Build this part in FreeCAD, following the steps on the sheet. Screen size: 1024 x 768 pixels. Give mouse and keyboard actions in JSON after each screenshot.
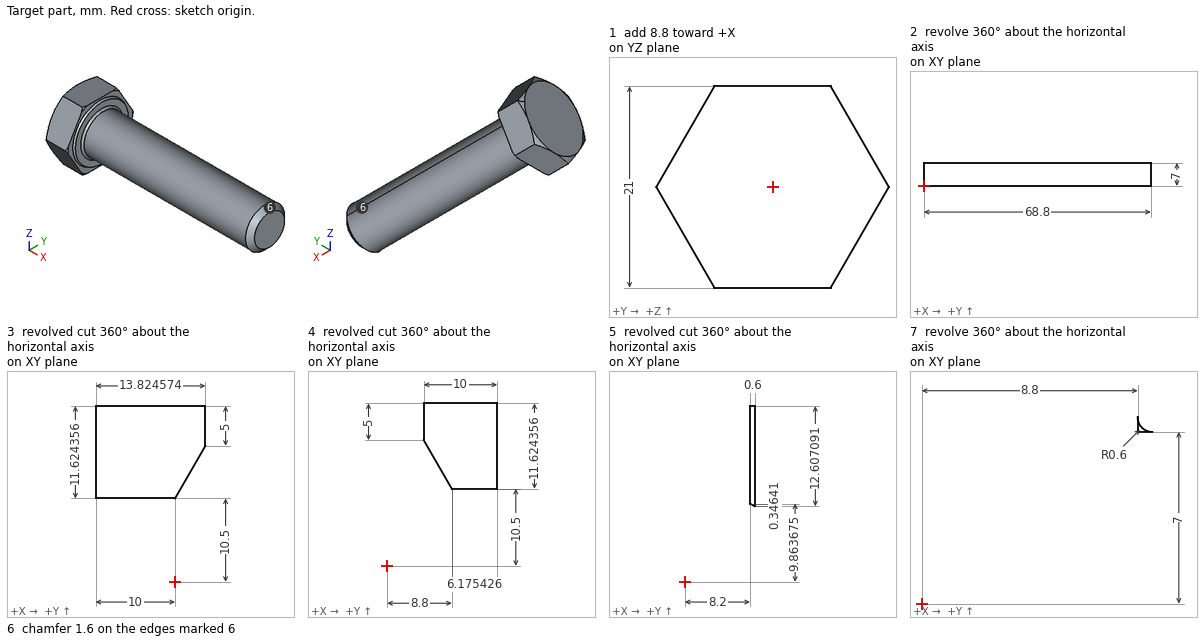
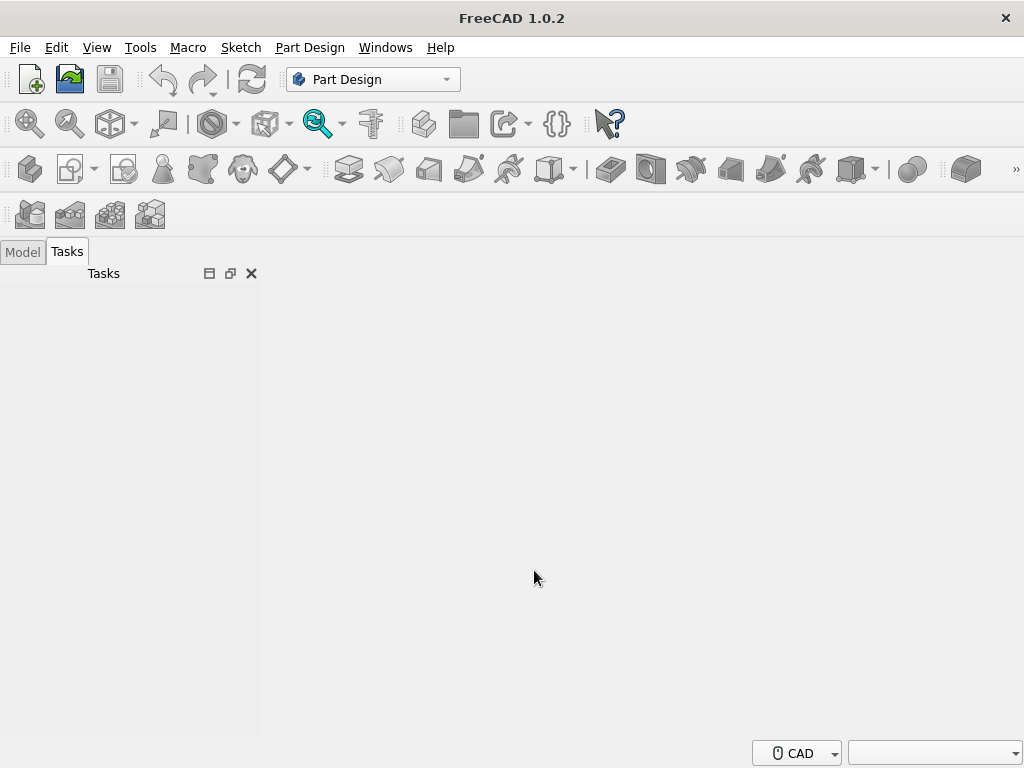
{"action": "left_click", "coordinate": [30, 80]}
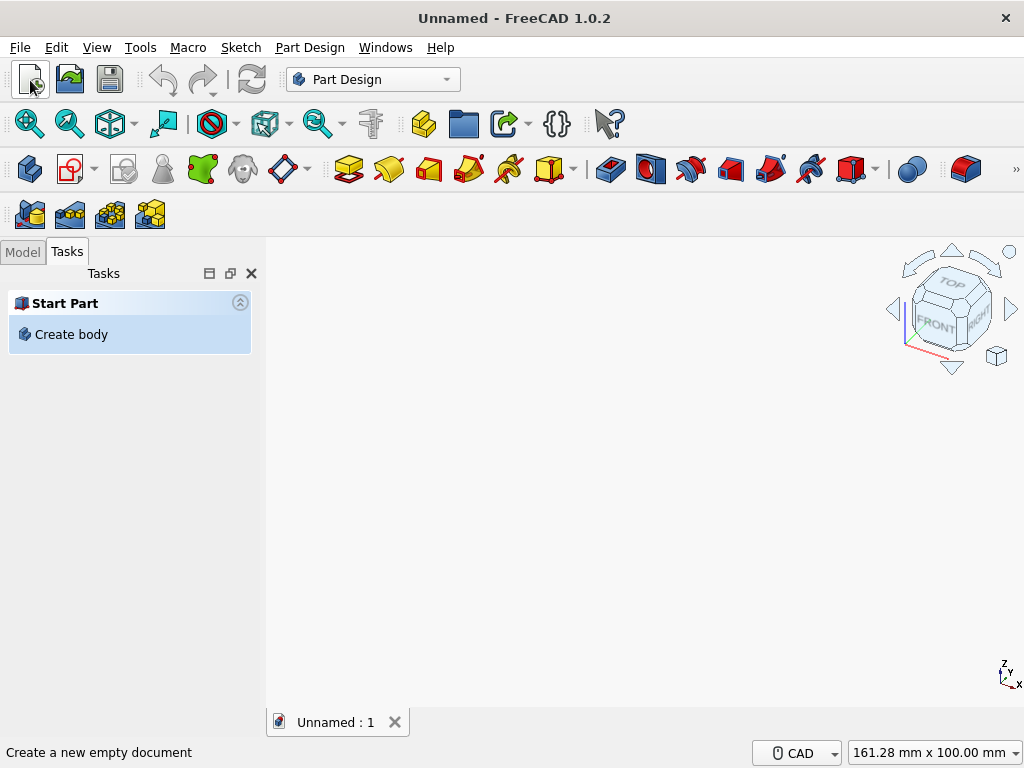
{"action": "left_click", "coordinate": [70, 170]}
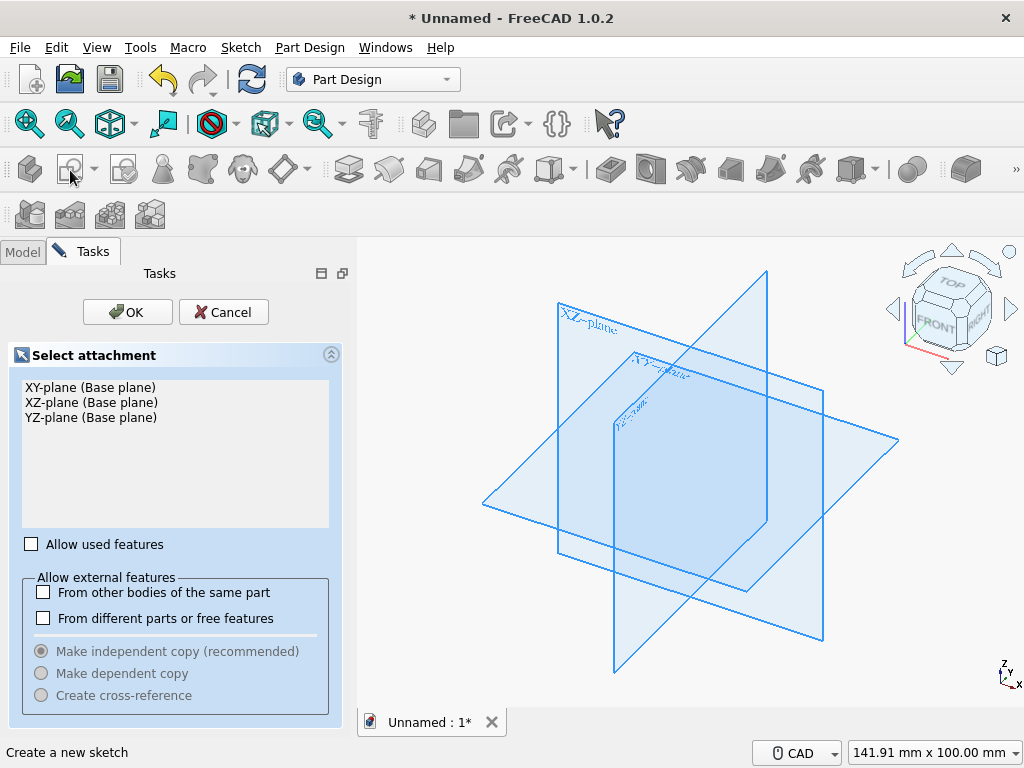
{"action": "left_click", "coordinate": [82, 418]}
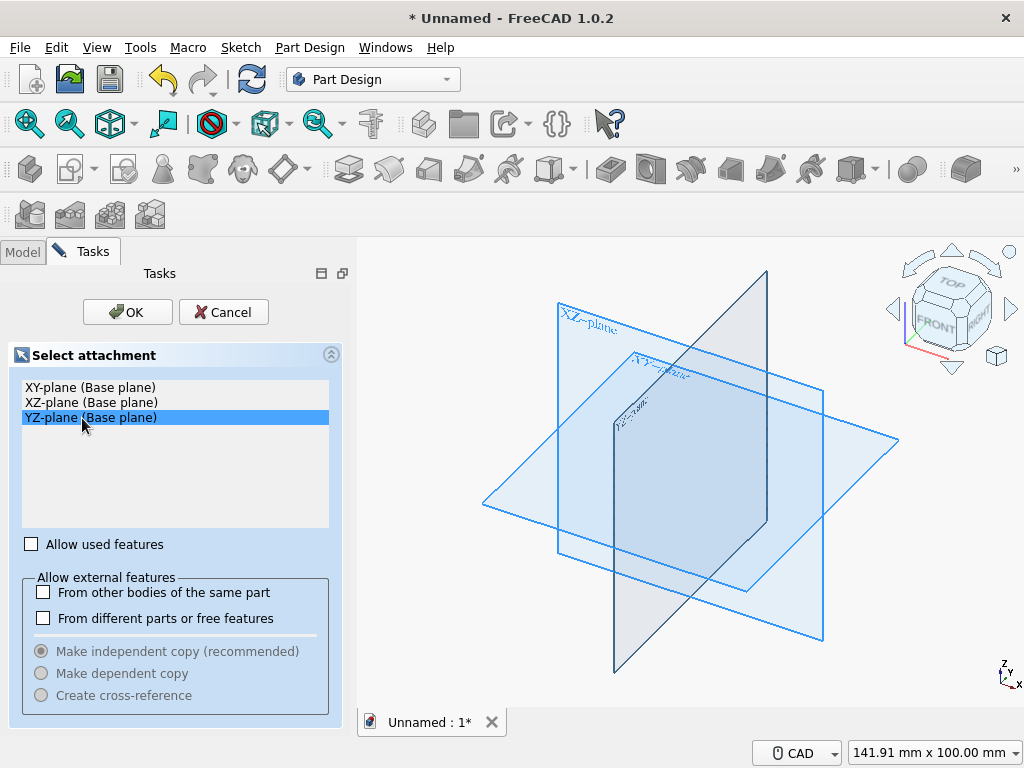
{"action": "left_click", "coordinate": [128, 312]}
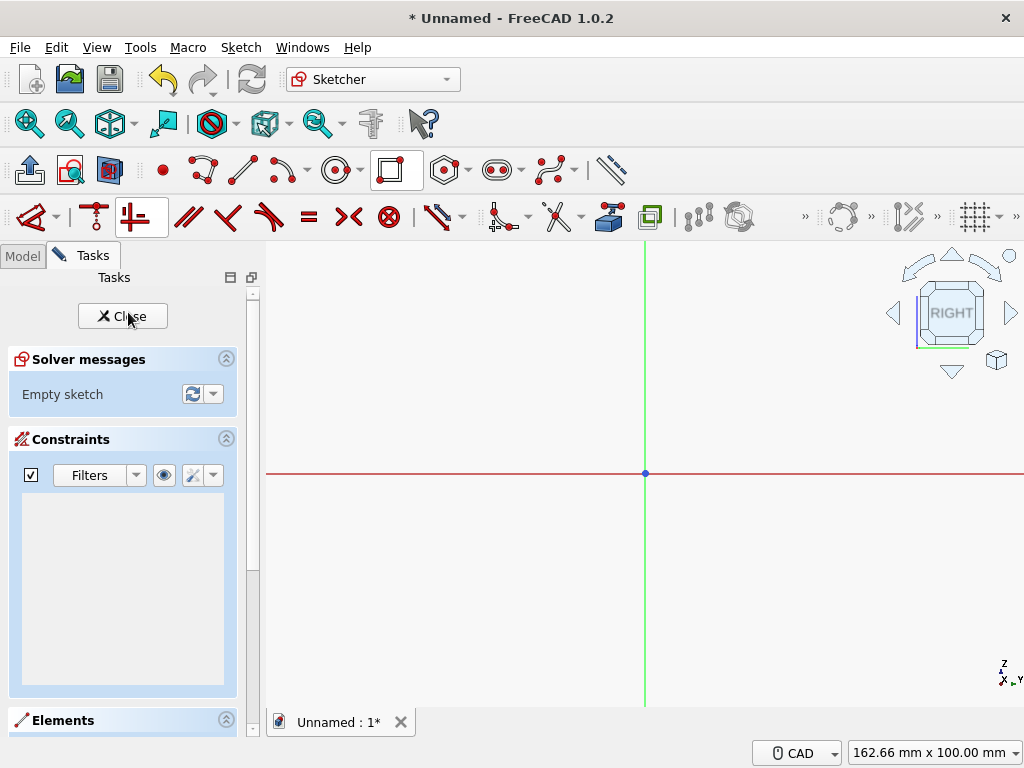
{"action": "scroll", "coordinate": [685, 474], "scroll_direction": "up", "scroll_amount": 5}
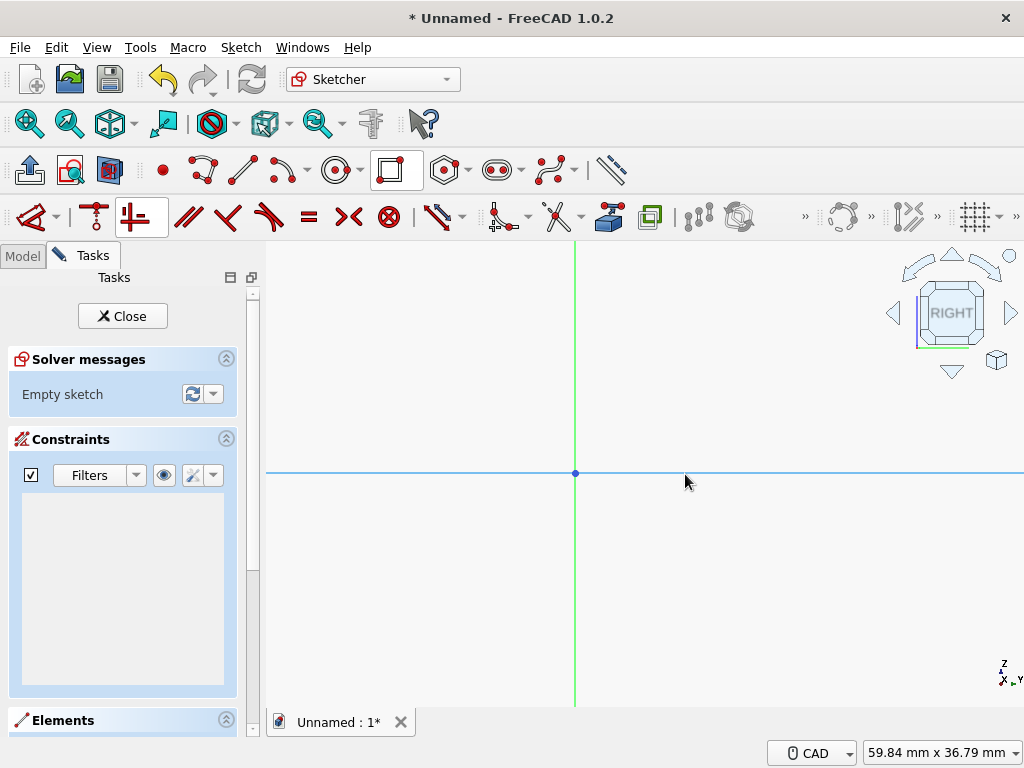
{"action": "left_click", "coordinate": [444, 170]}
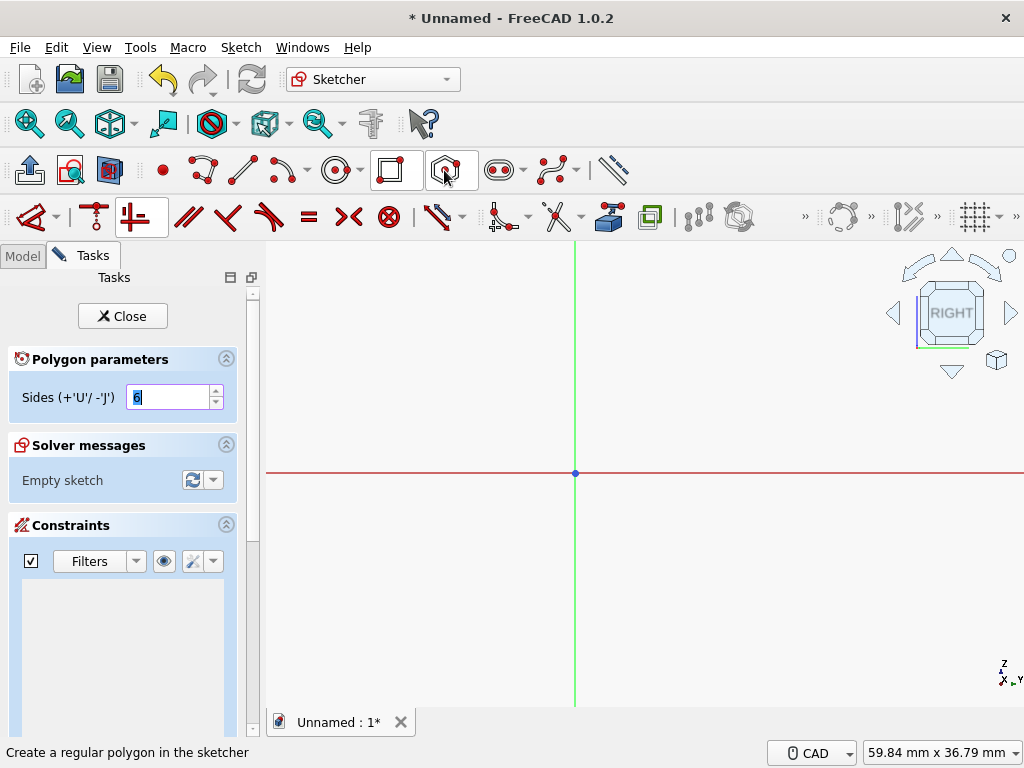
{"action": "left_click", "coordinate": [575, 473]}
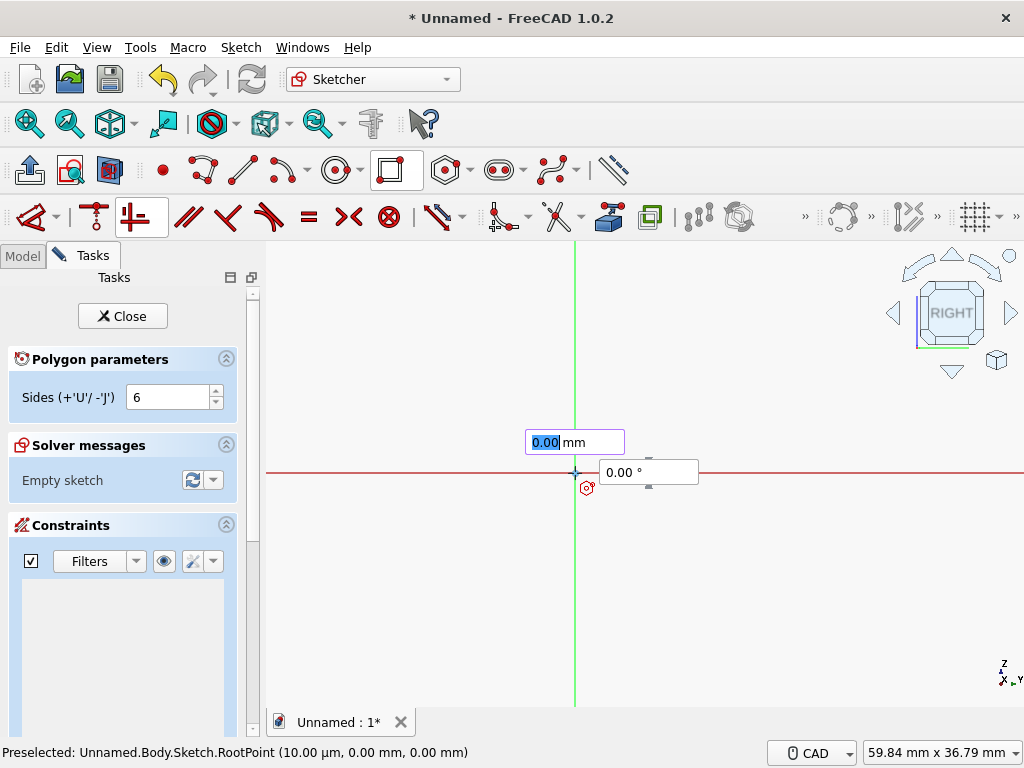
{"action": "left_click", "coordinate": [729, 473]}
{"action": "right_click", "coordinate": [729, 473]}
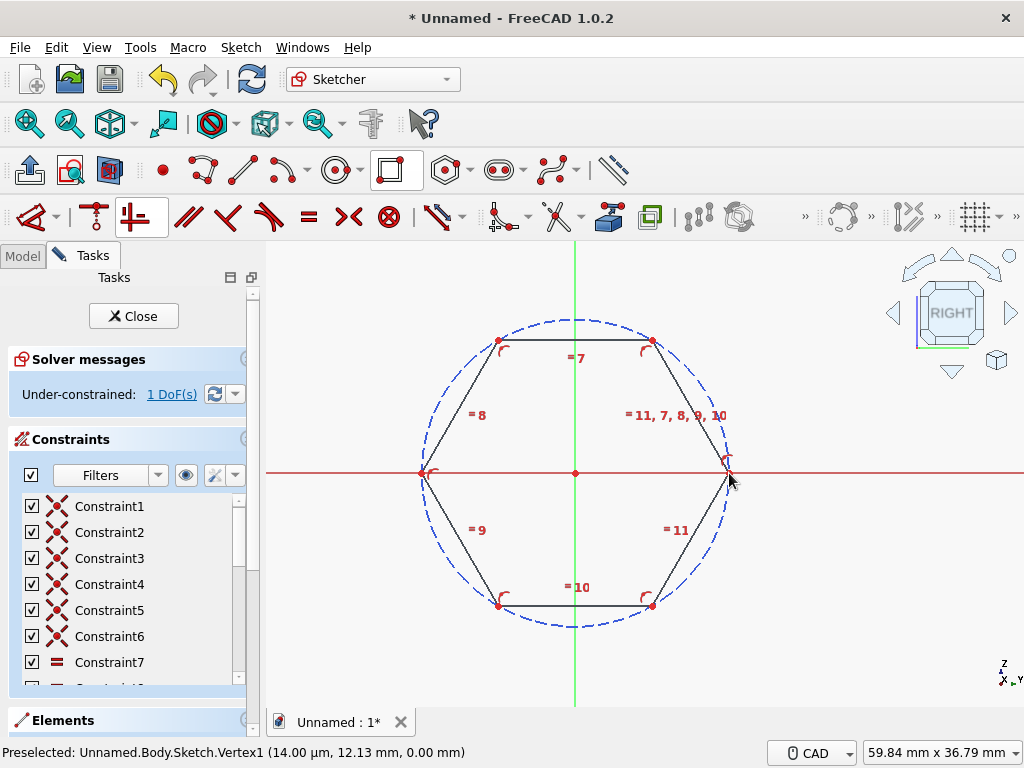
{"action": "left_click", "coordinate": [498, 606]}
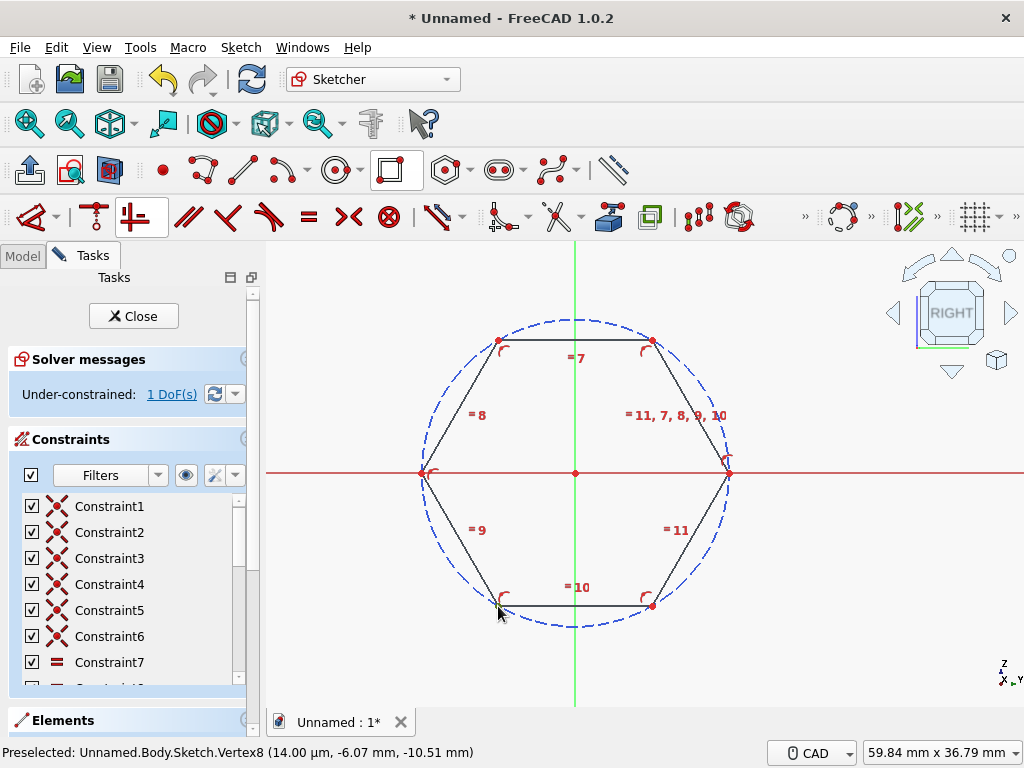
{"action": "left_click", "coordinate": [652, 340]}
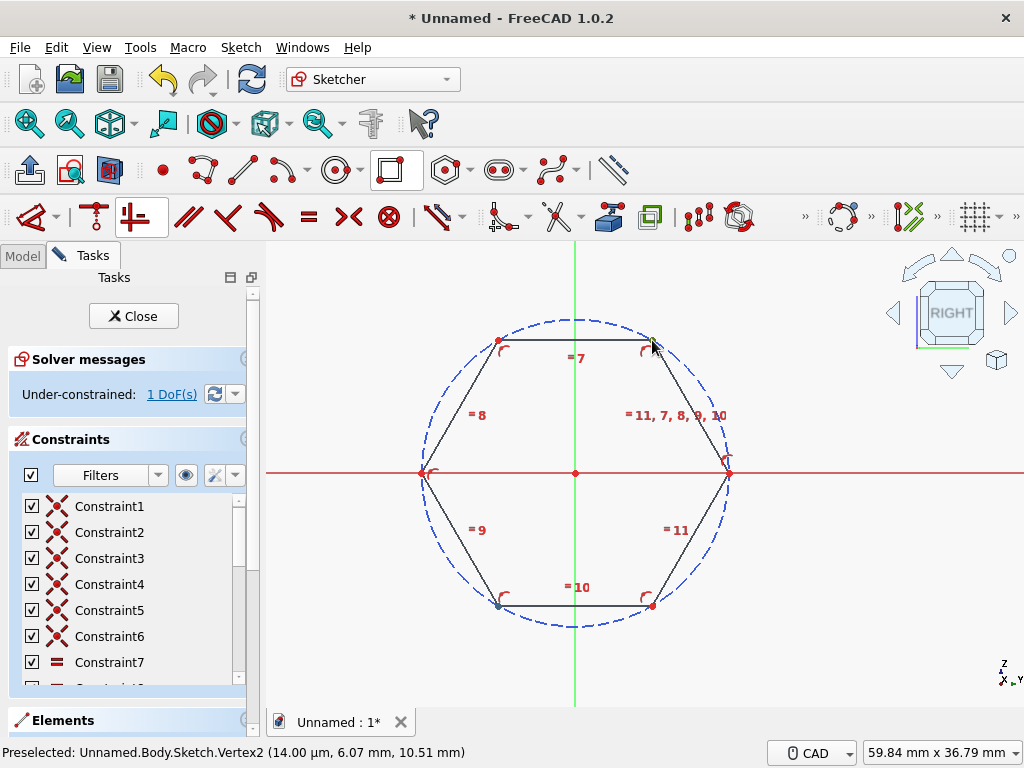
{"action": "key", "text": "i"}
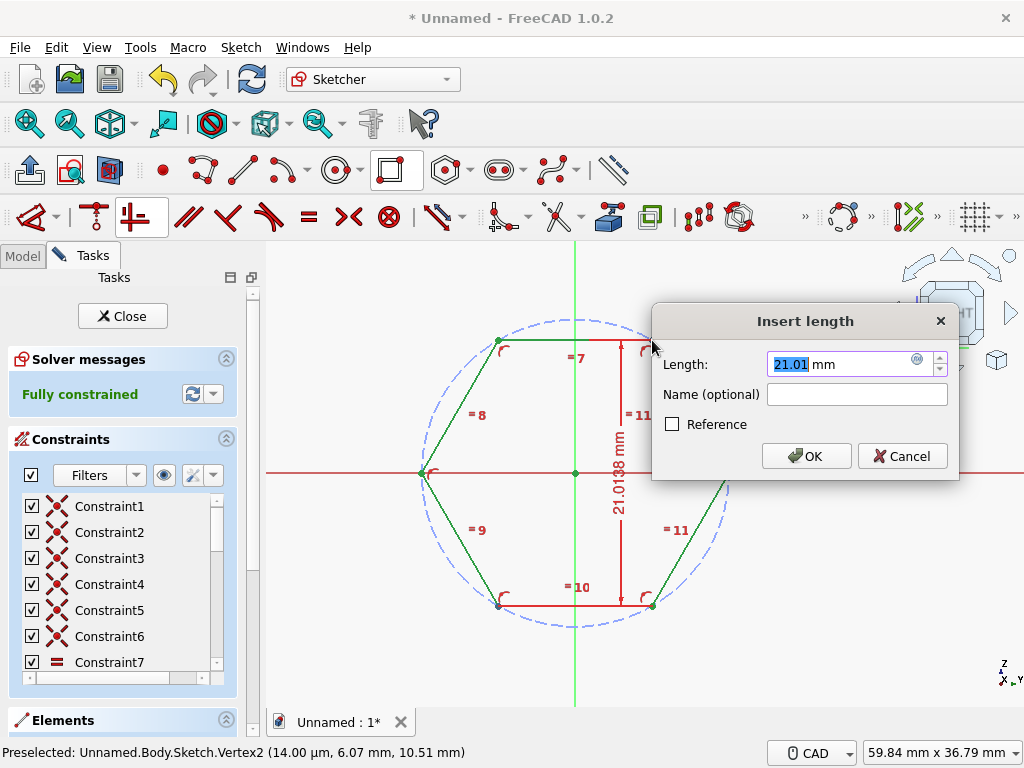
{"action": "type", "text": "21"}
{"action": "key", "text": "Return"}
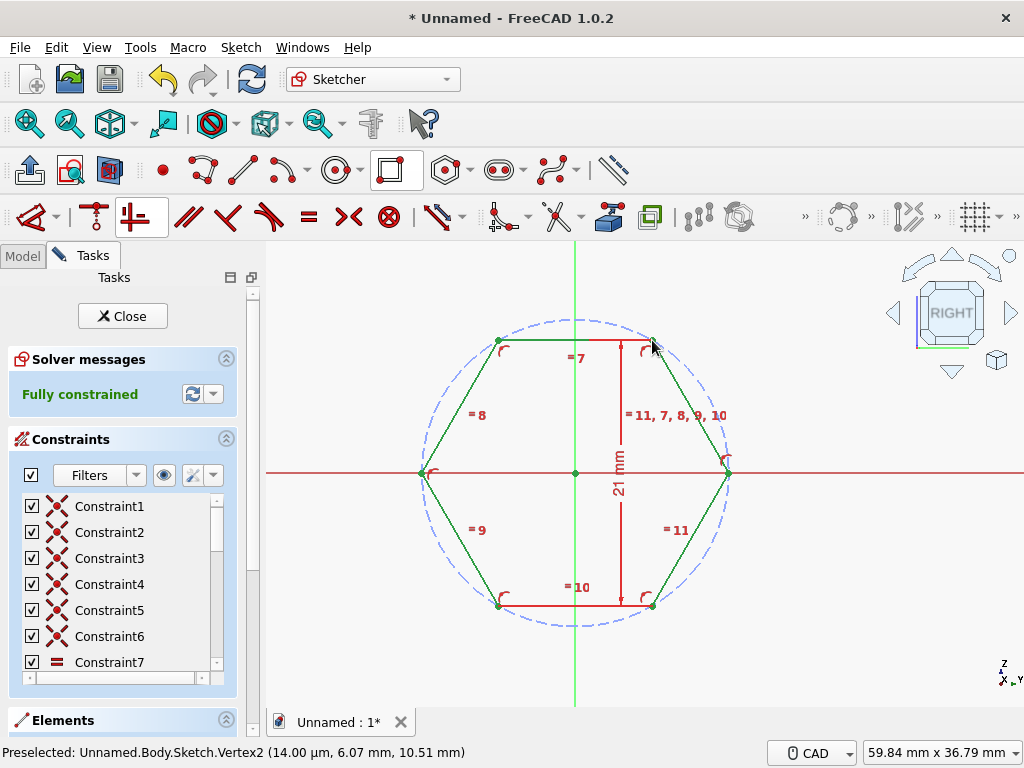
{"action": "left_click", "coordinate": [123, 316]}